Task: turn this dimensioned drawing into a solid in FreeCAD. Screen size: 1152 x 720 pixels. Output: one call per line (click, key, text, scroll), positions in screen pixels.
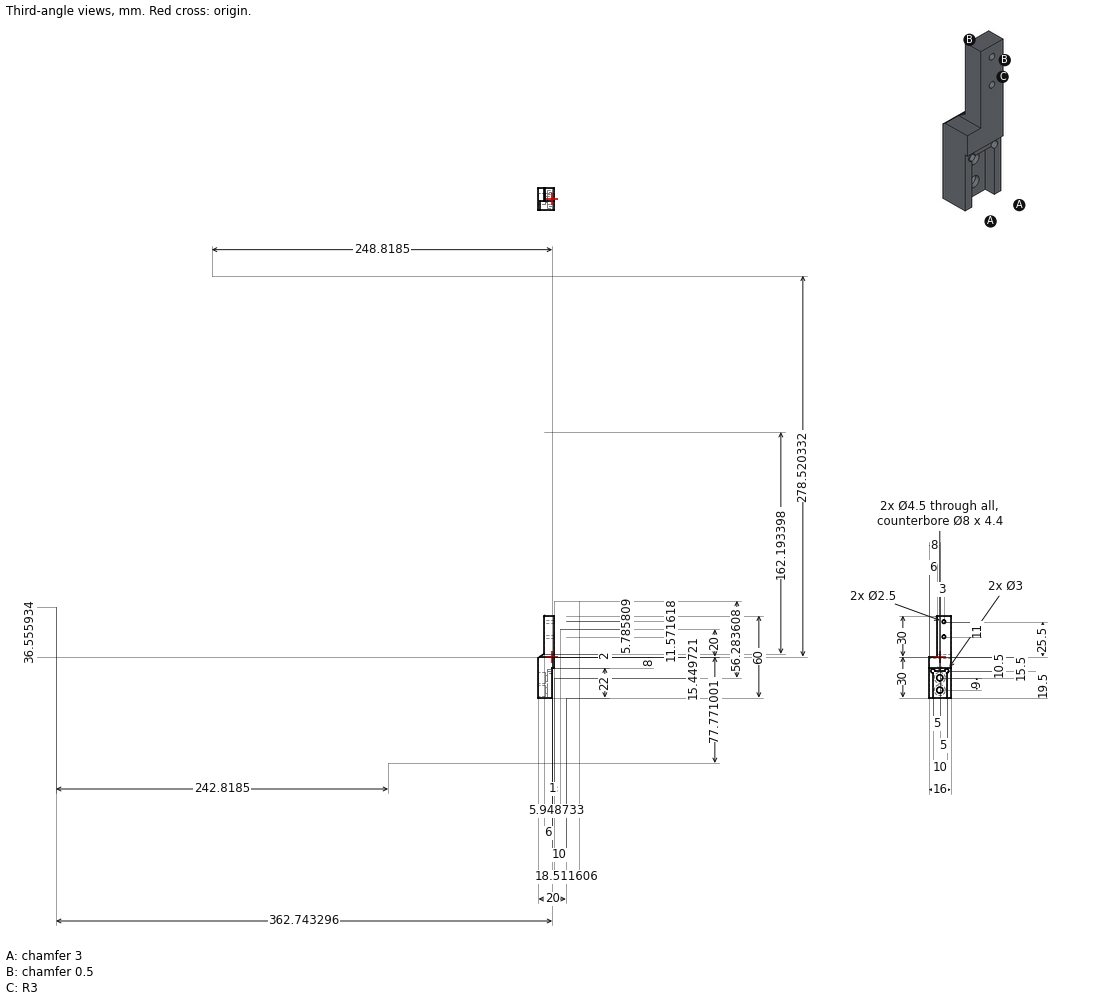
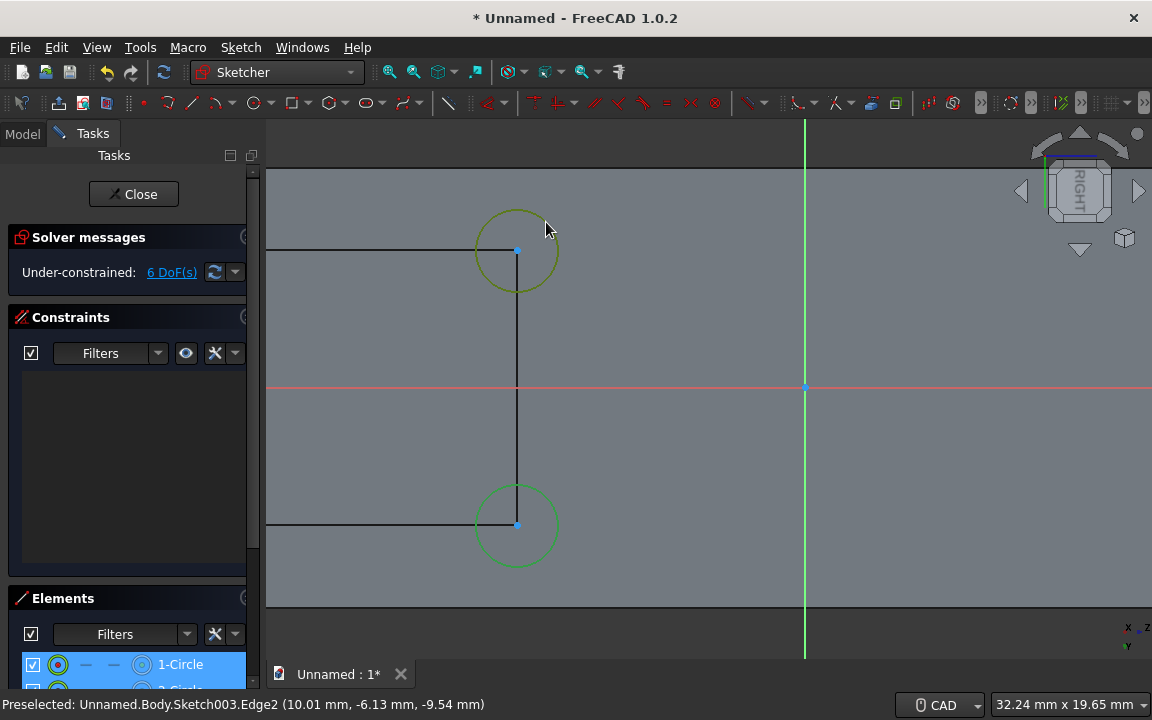
key(e)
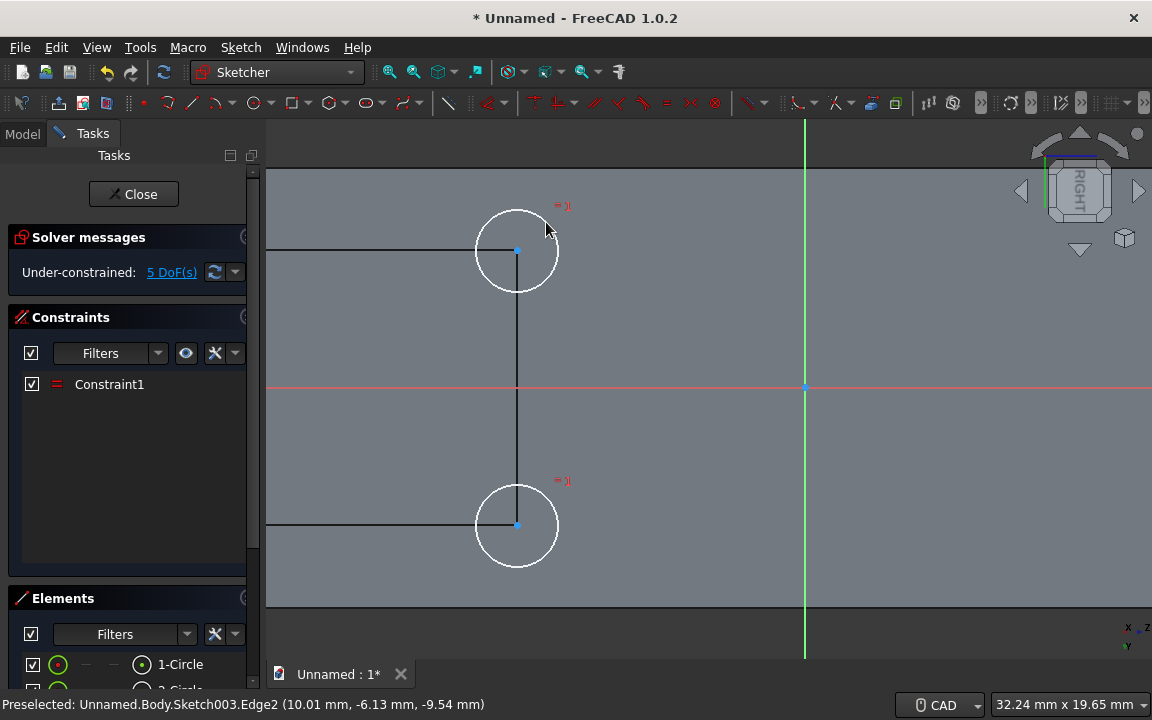
click(517, 526)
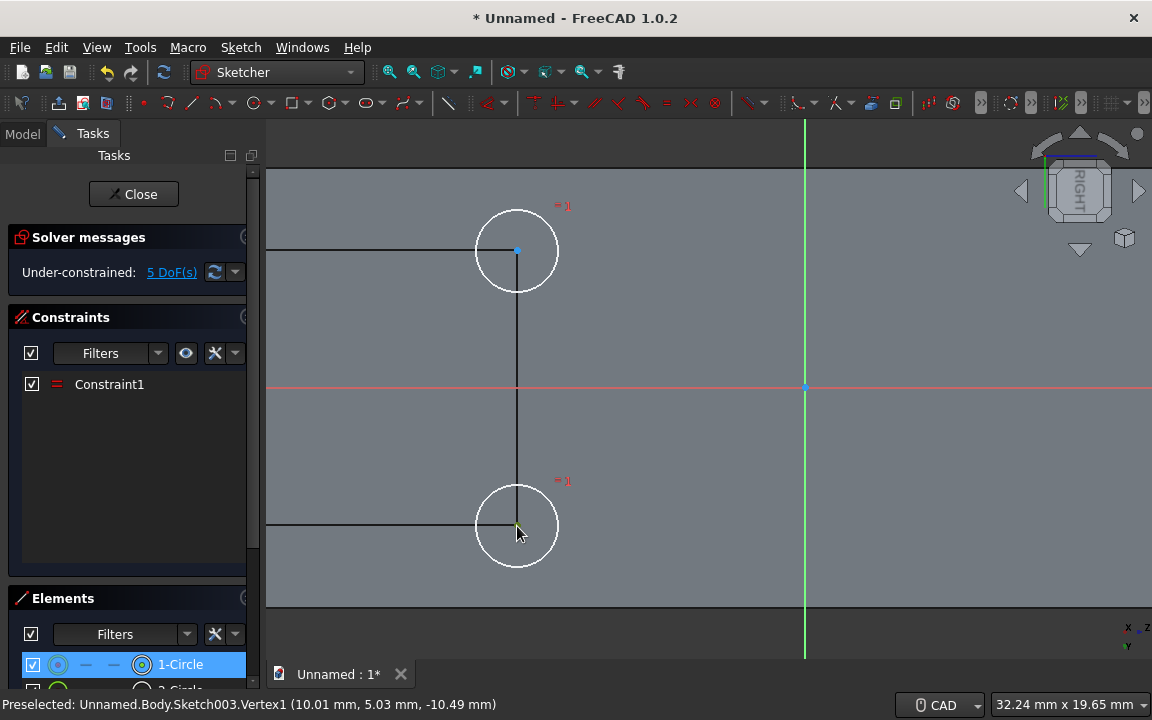
click(517, 251)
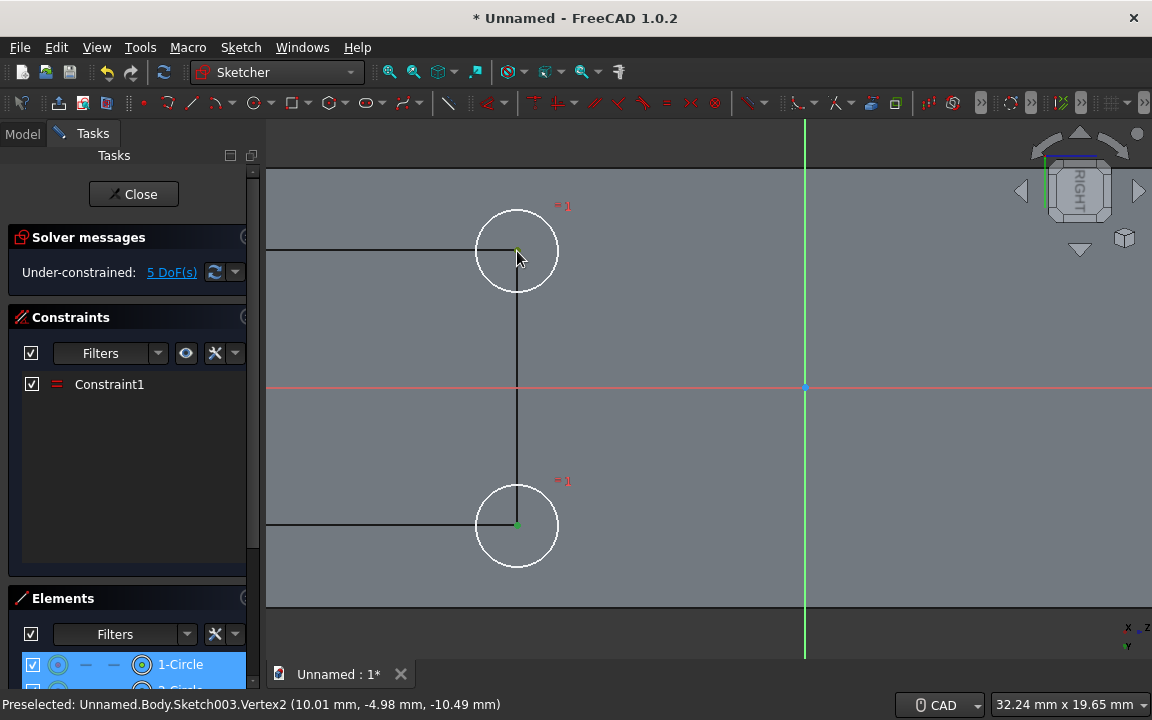
key(v)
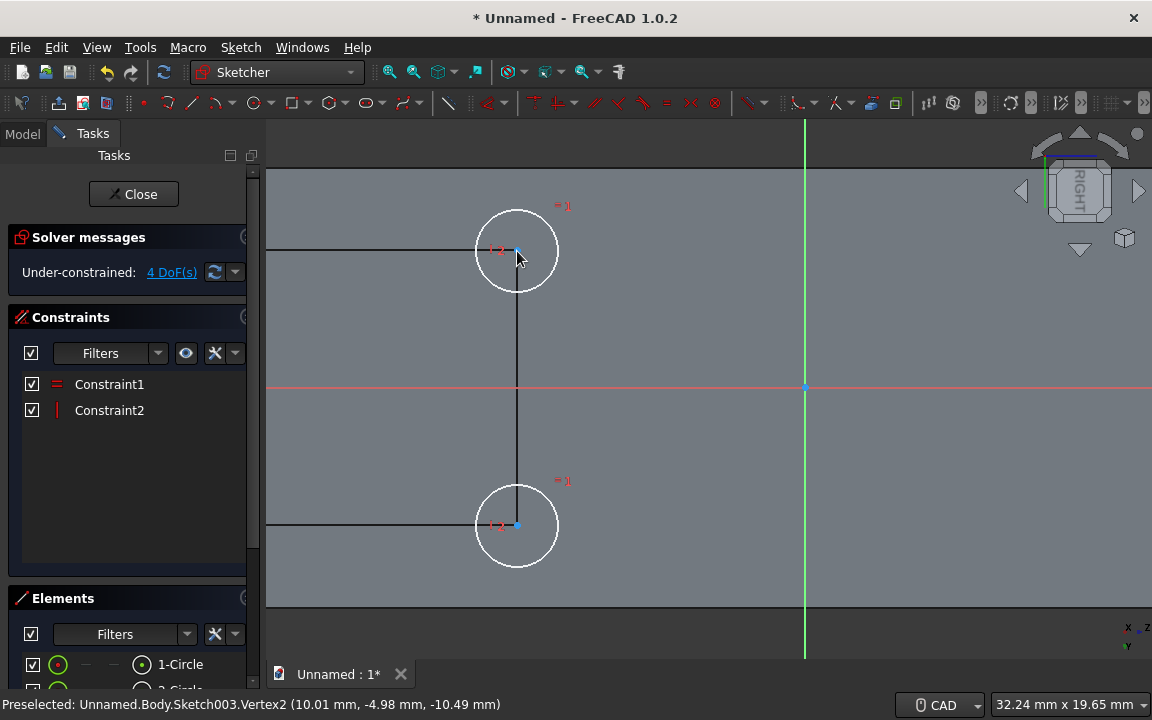
key(d)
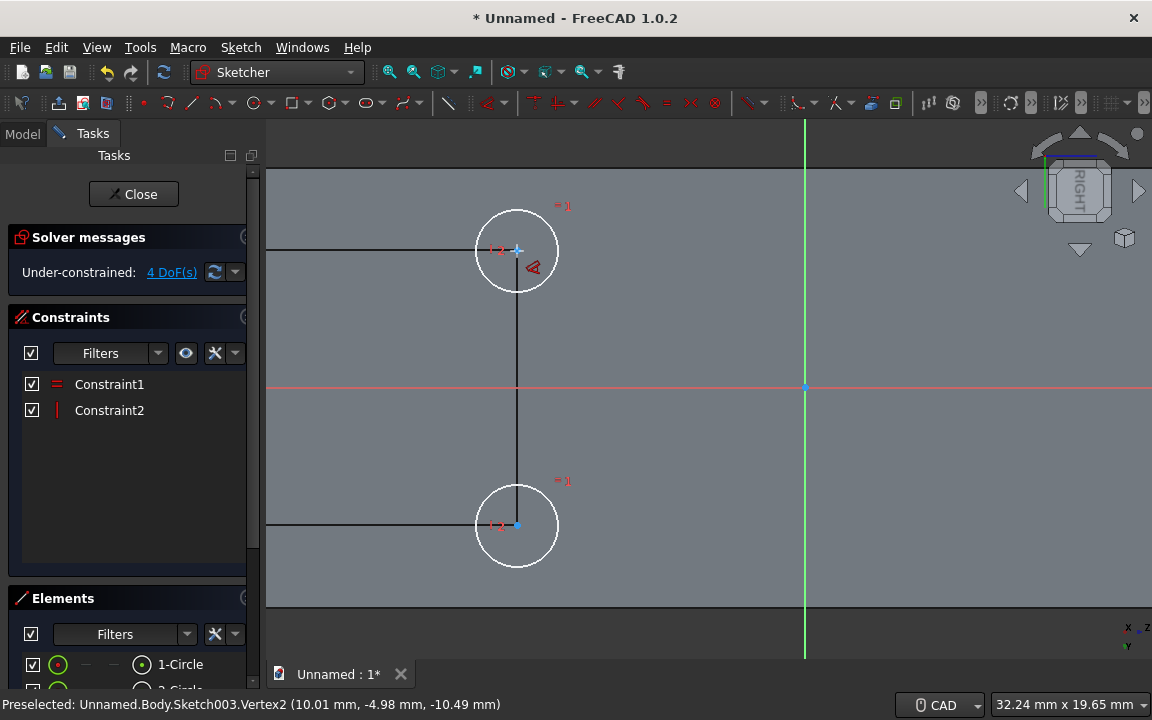
click(546, 497)
click(569, 474)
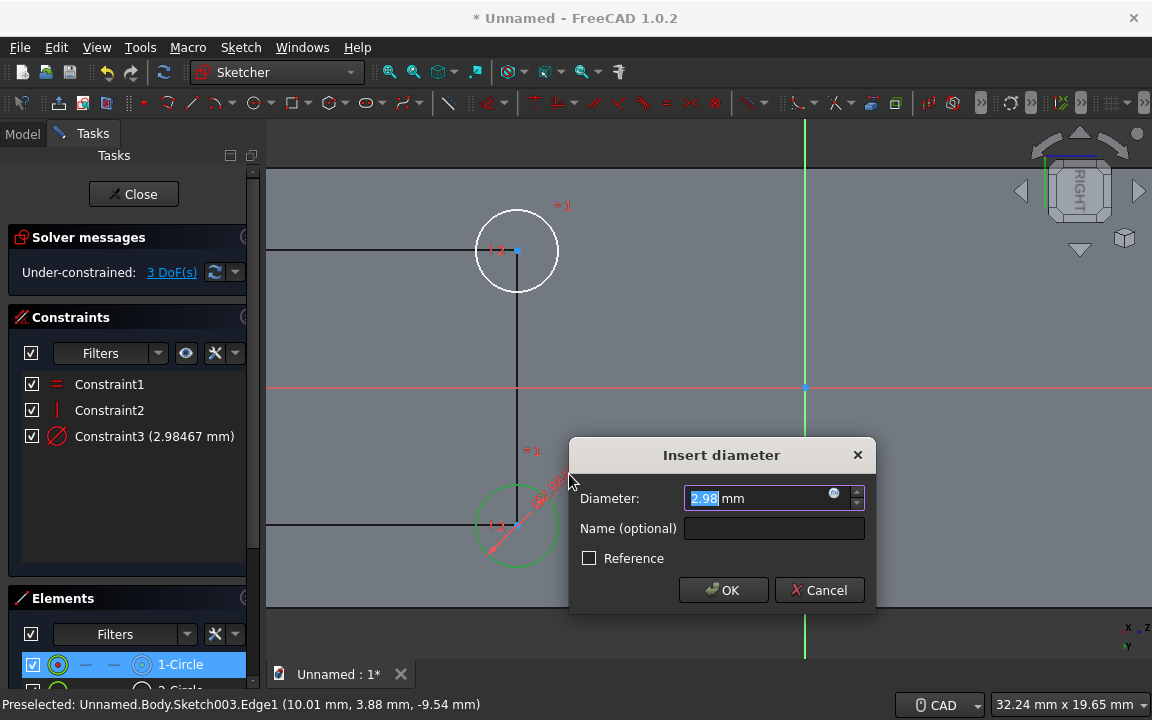
text(3)
key(Return)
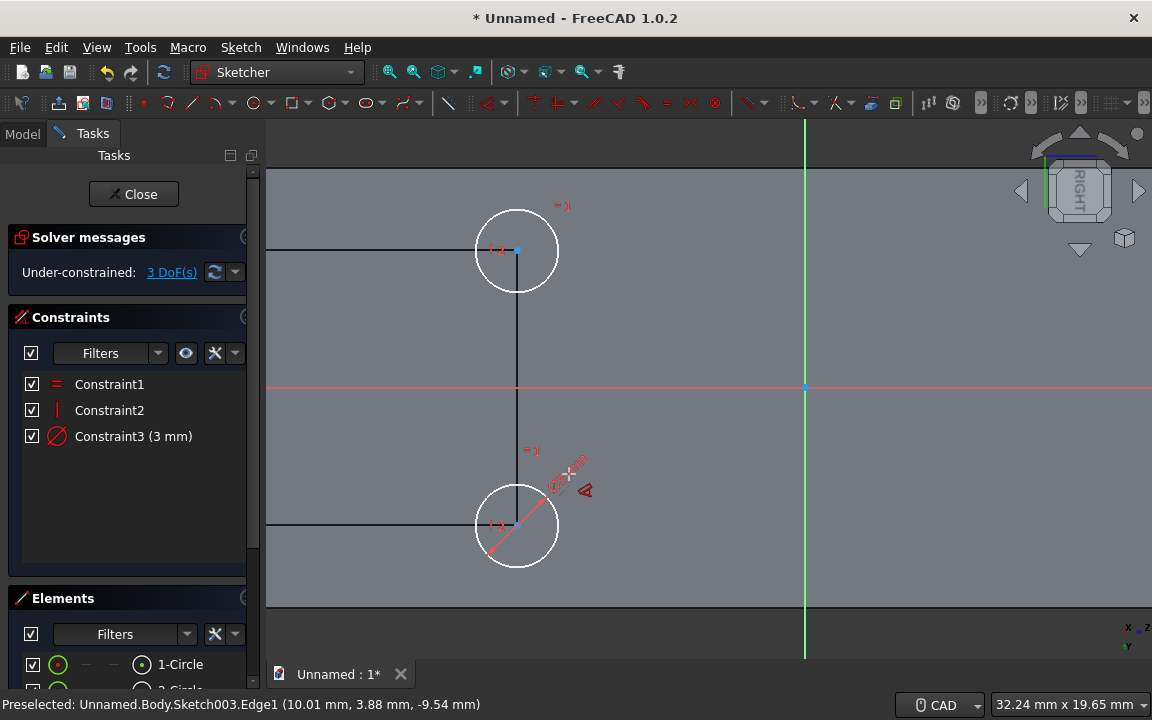
click(517, 526)
click(839, 457)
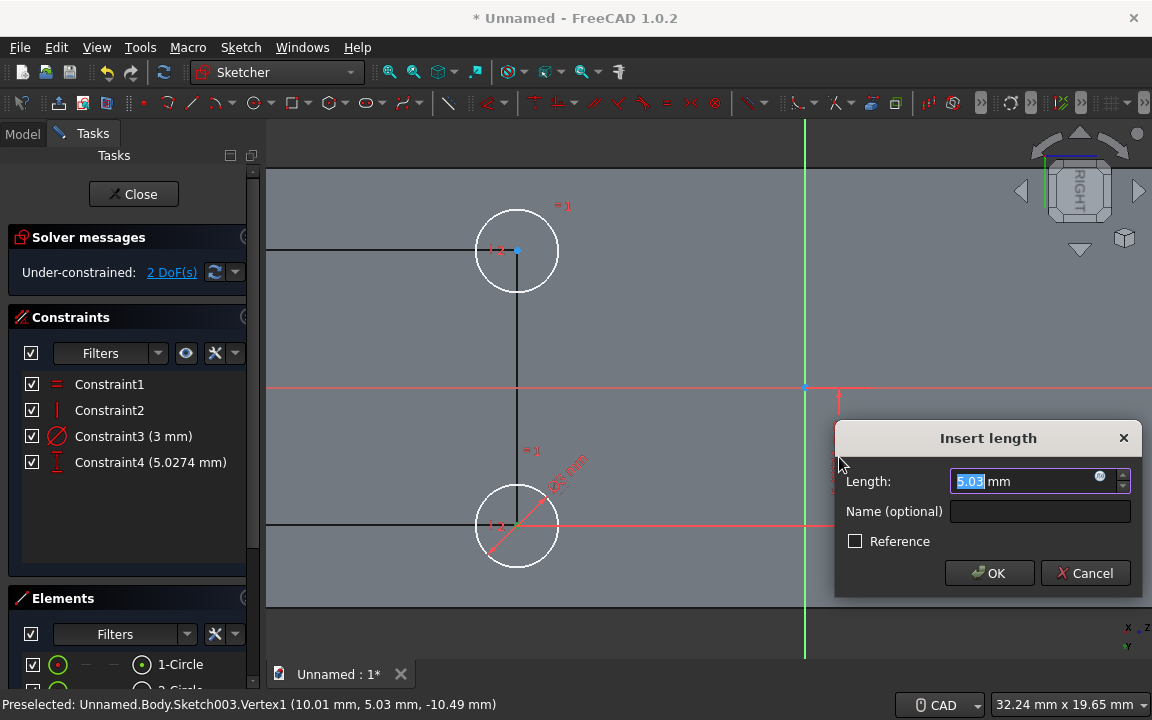
text(5)
key(Return)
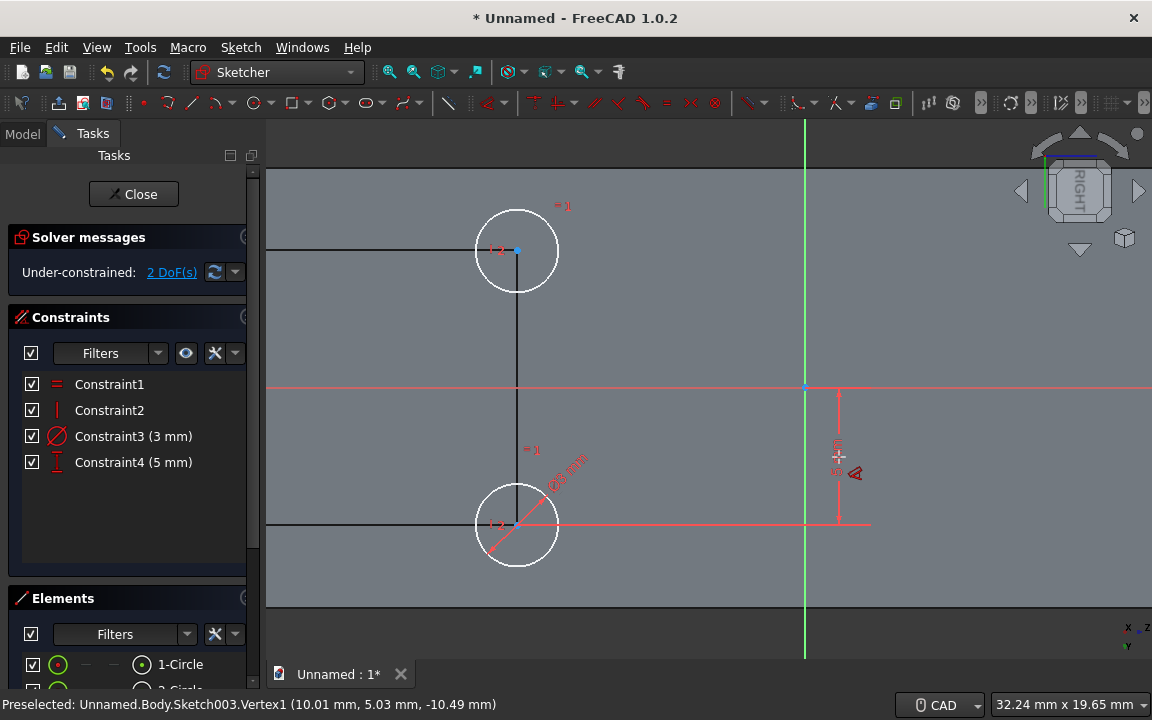
click(517, 251)
click(839, 319)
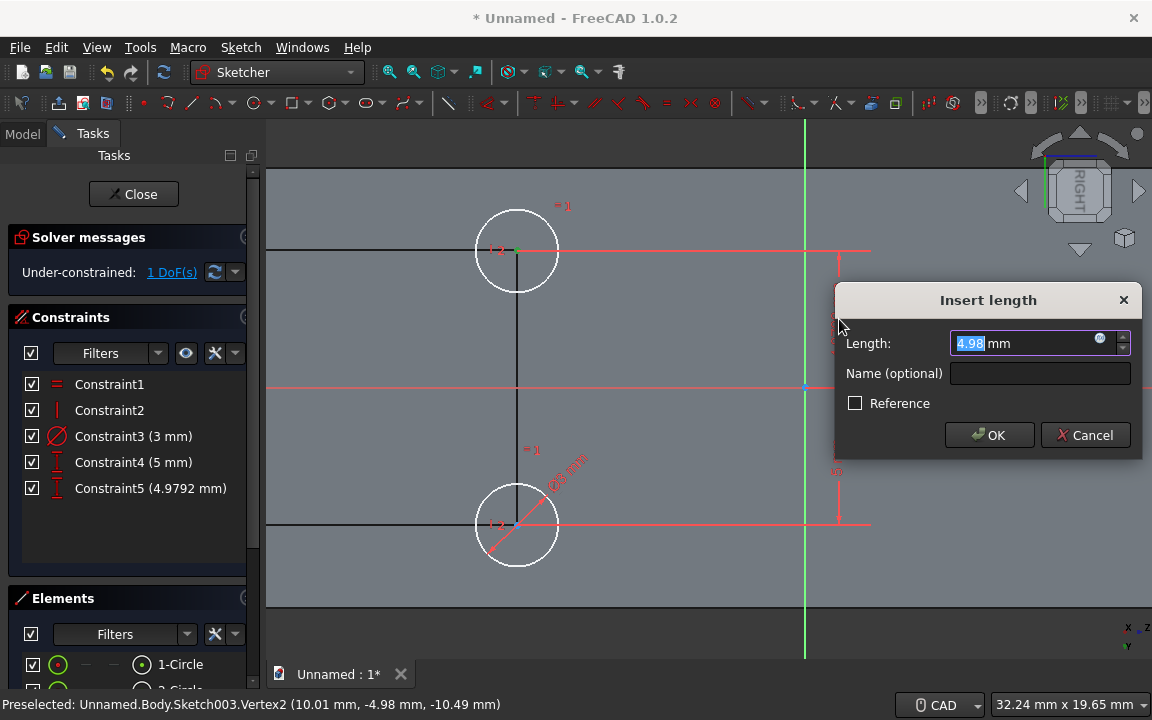
text(5)
key(Return)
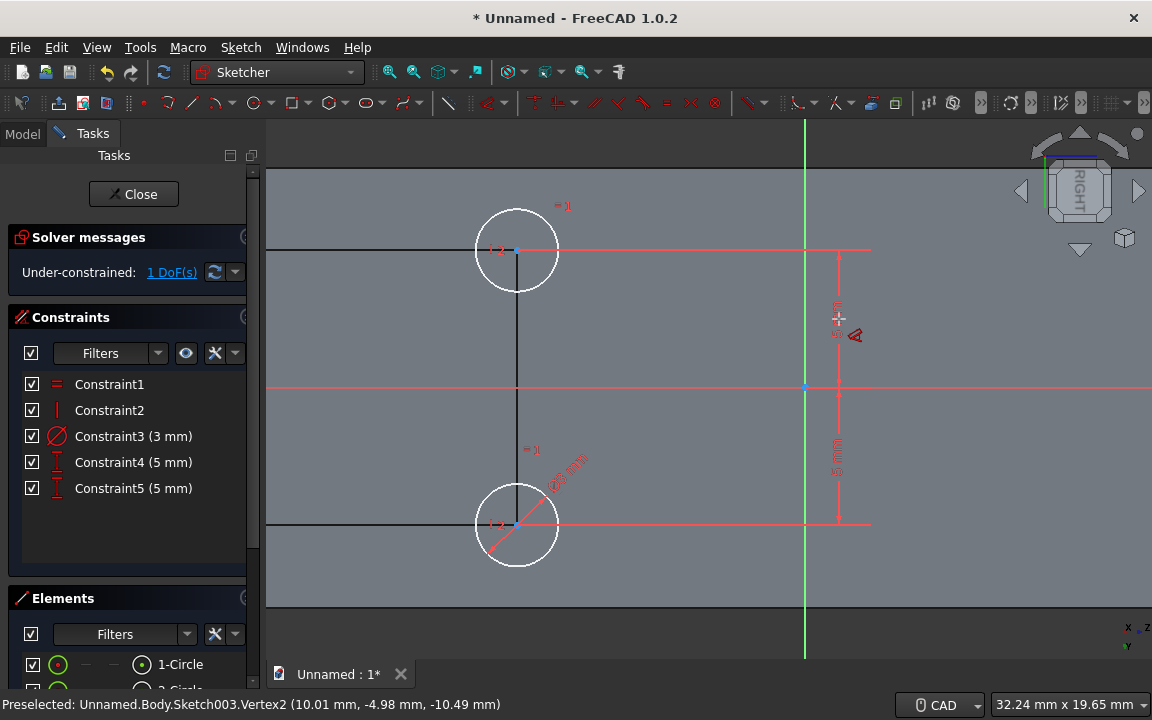
click(517, 525)
click(661, 559)